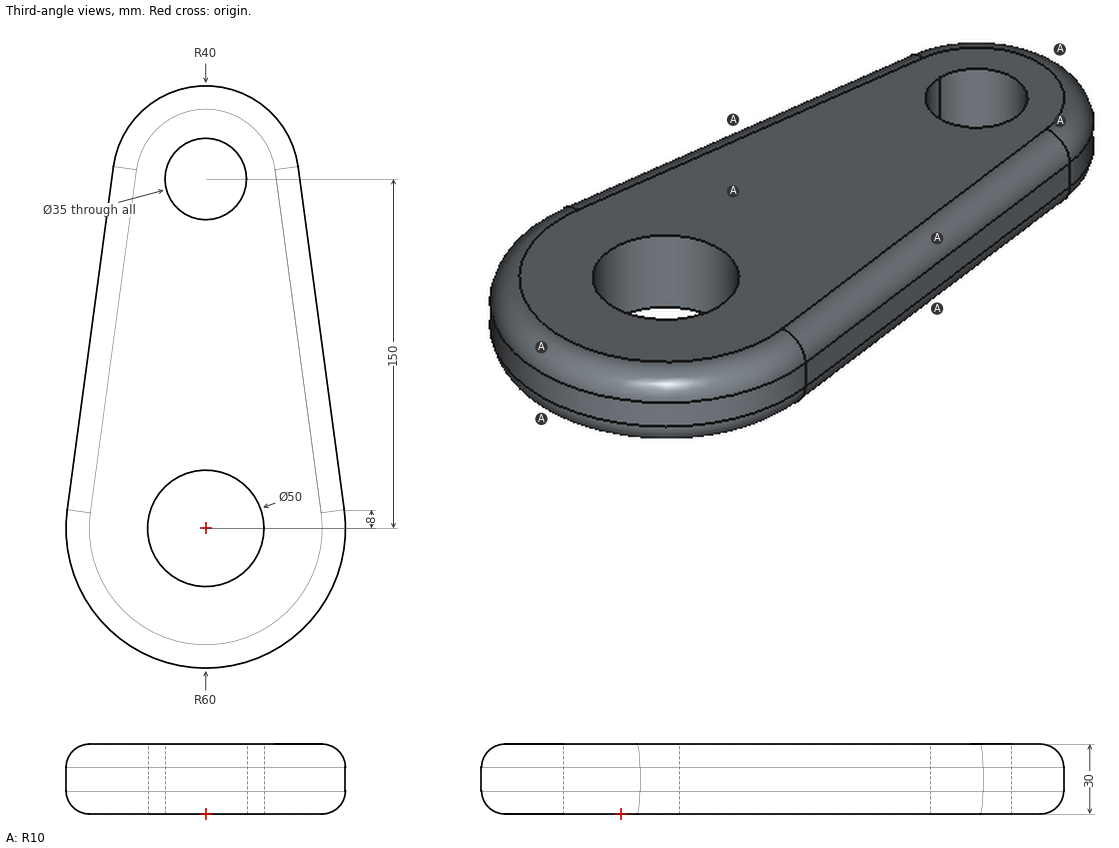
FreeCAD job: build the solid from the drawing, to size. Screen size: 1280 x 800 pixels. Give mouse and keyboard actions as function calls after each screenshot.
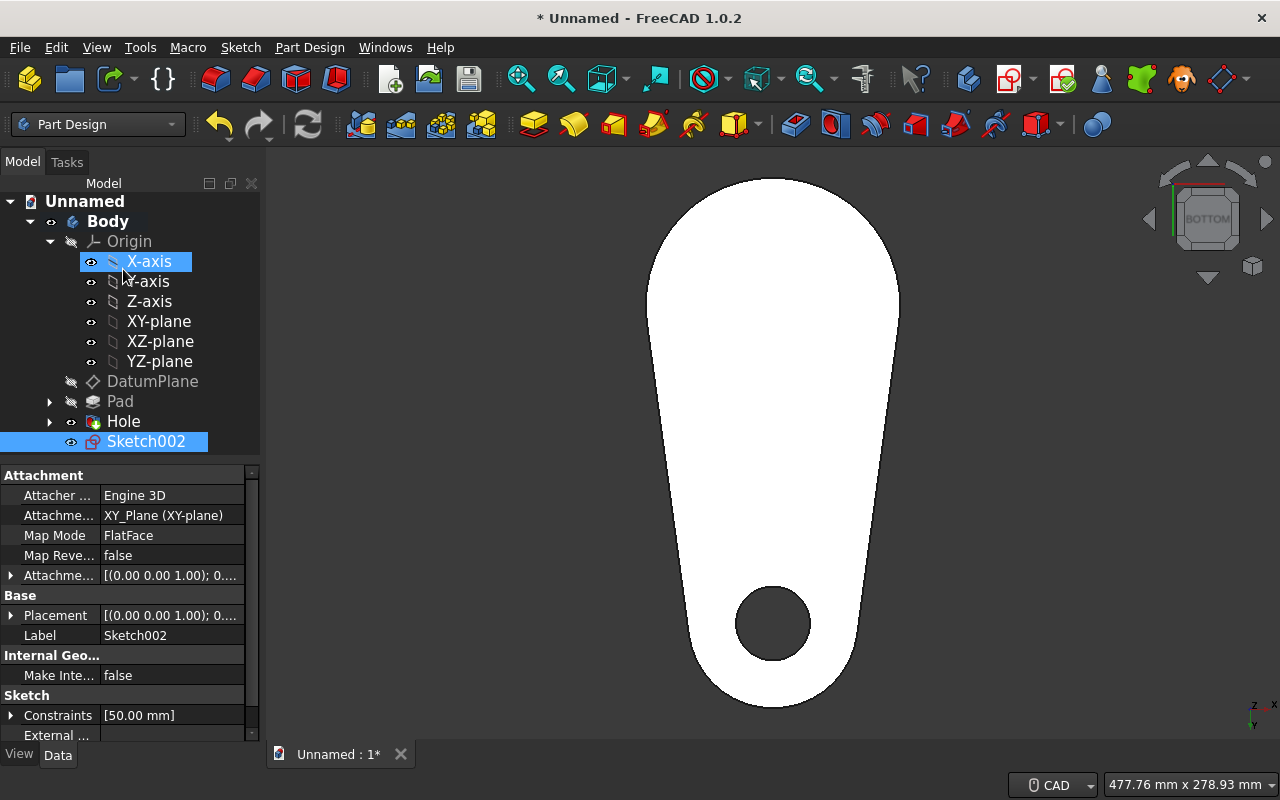
click(796, 124)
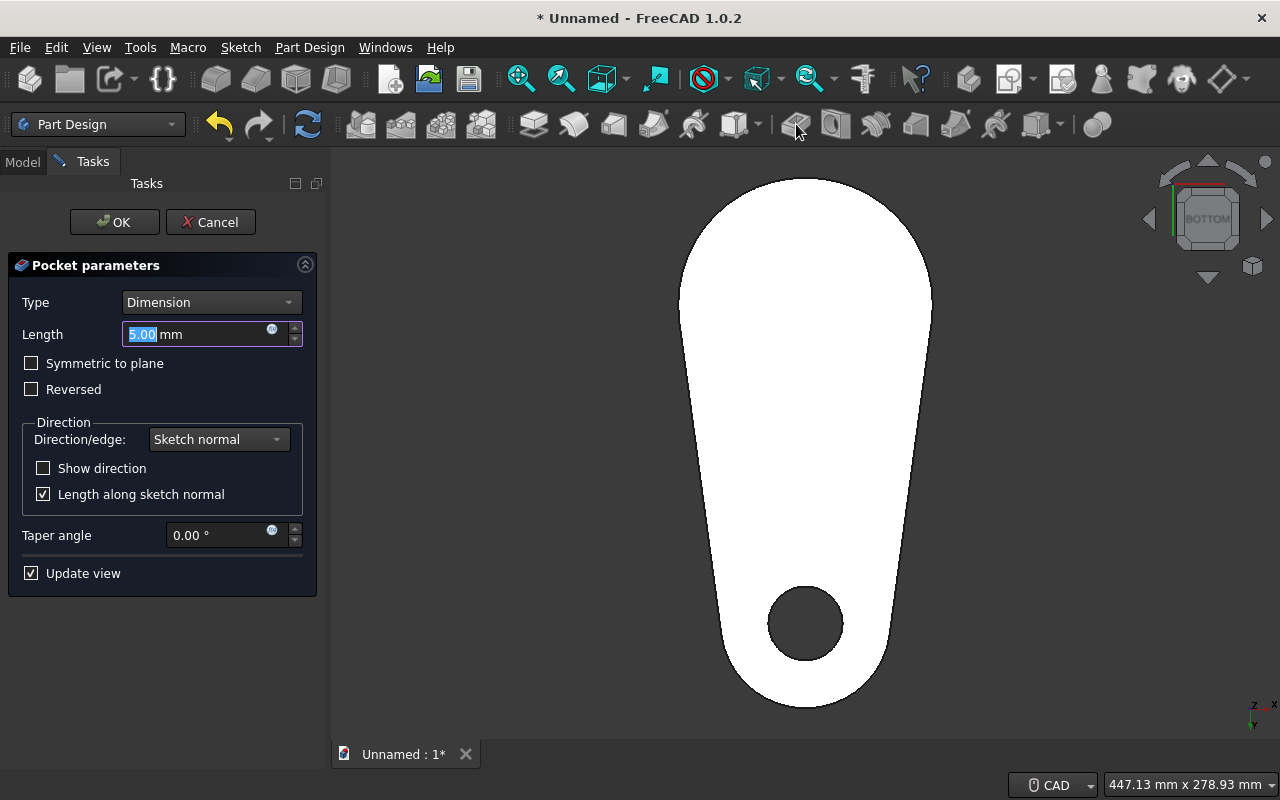
click(212, 302)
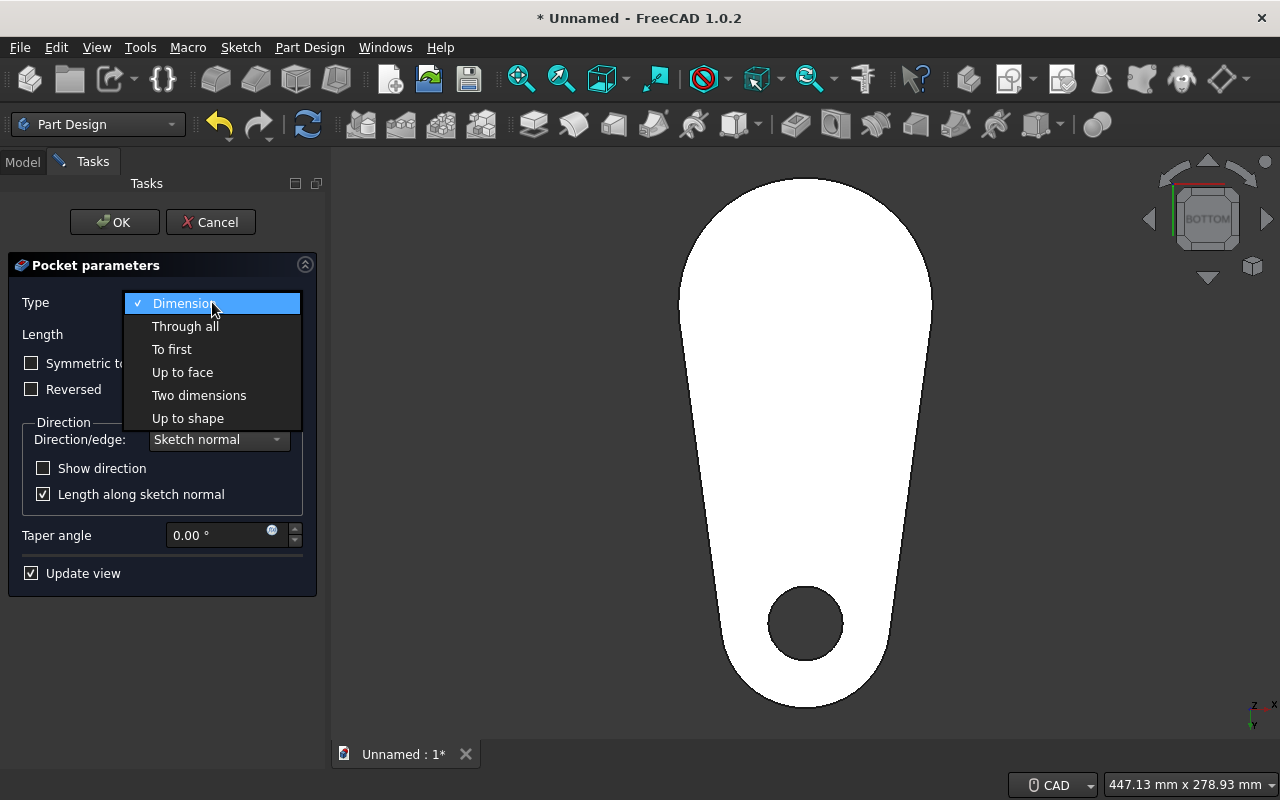
click(212, 326)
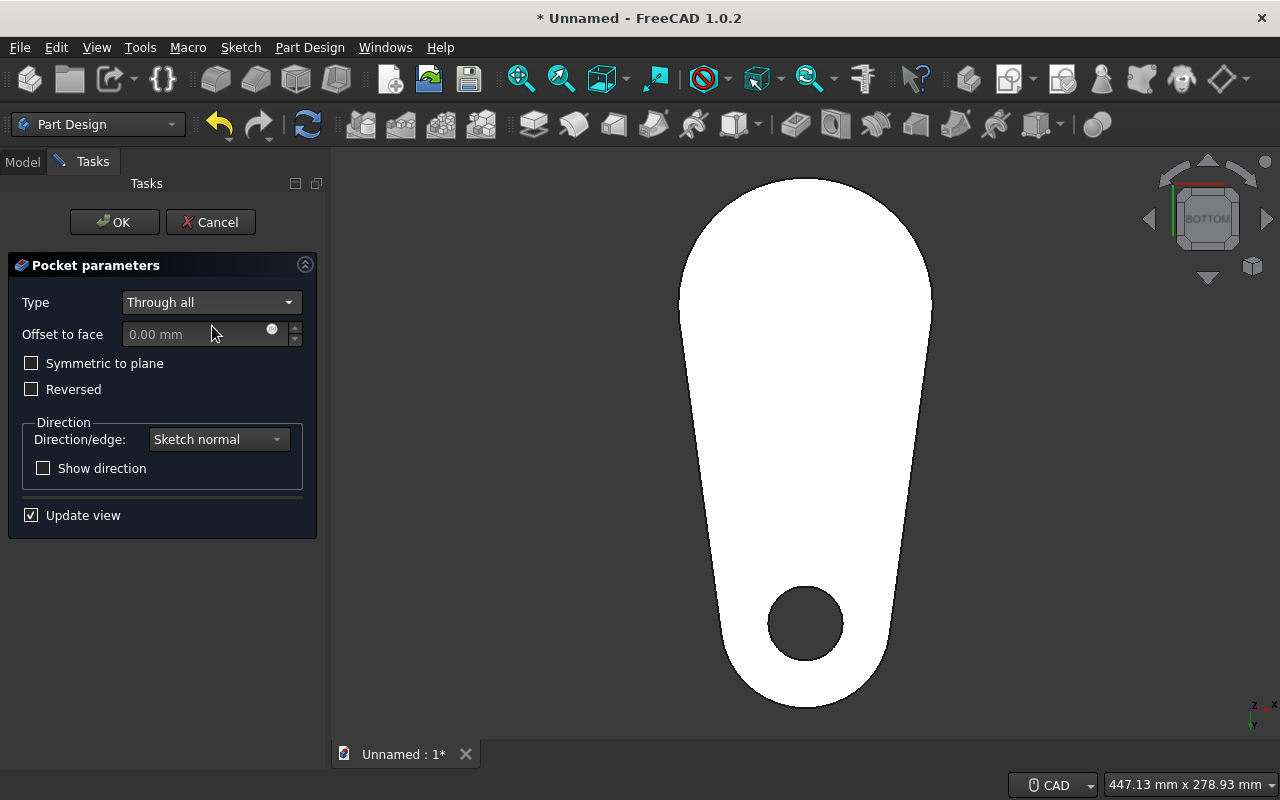
click(30, 389)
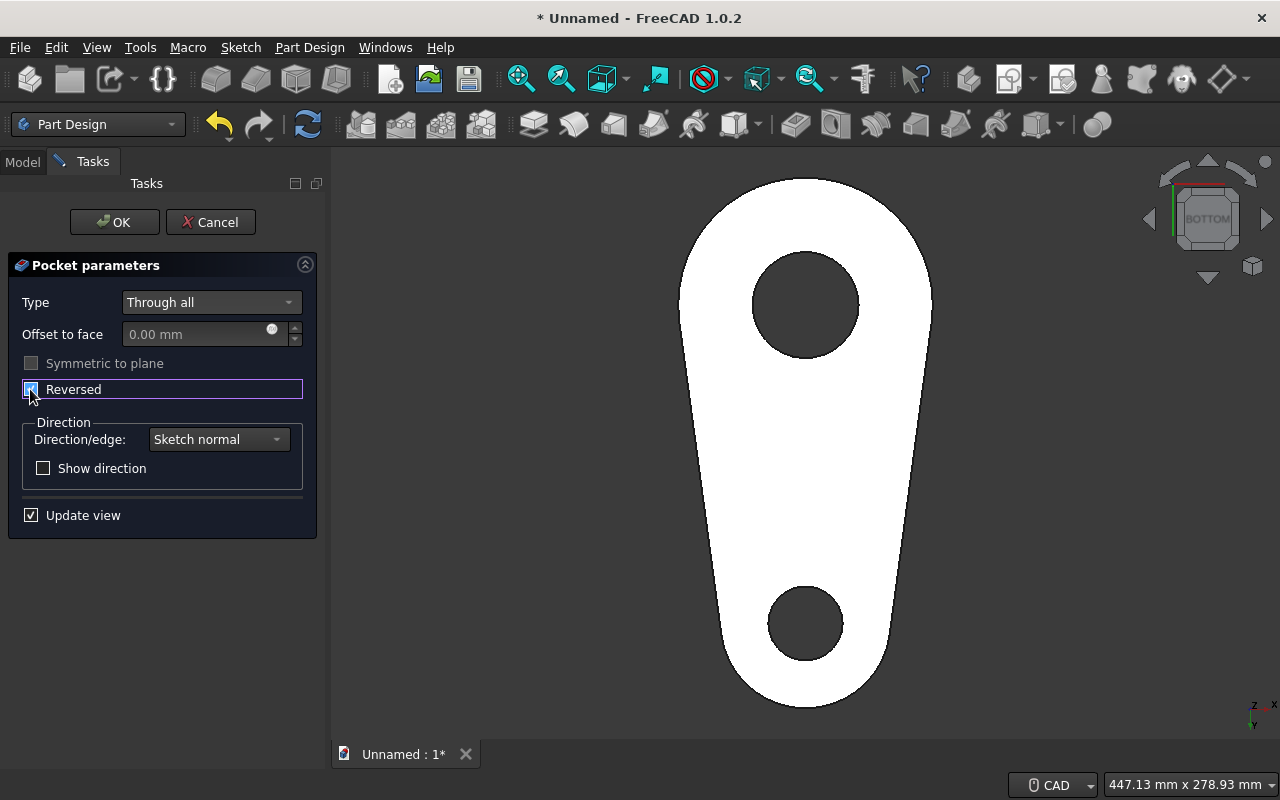
click(115, 222)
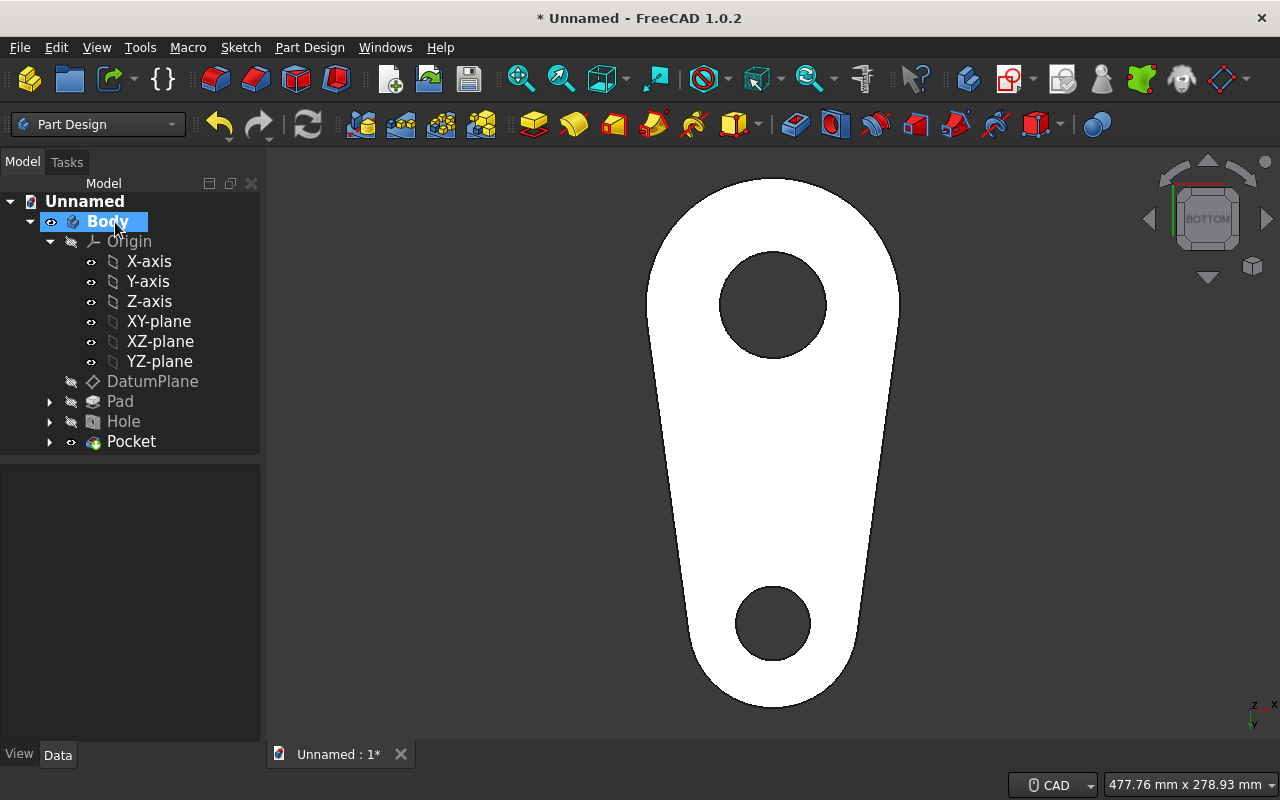
click(773, 707)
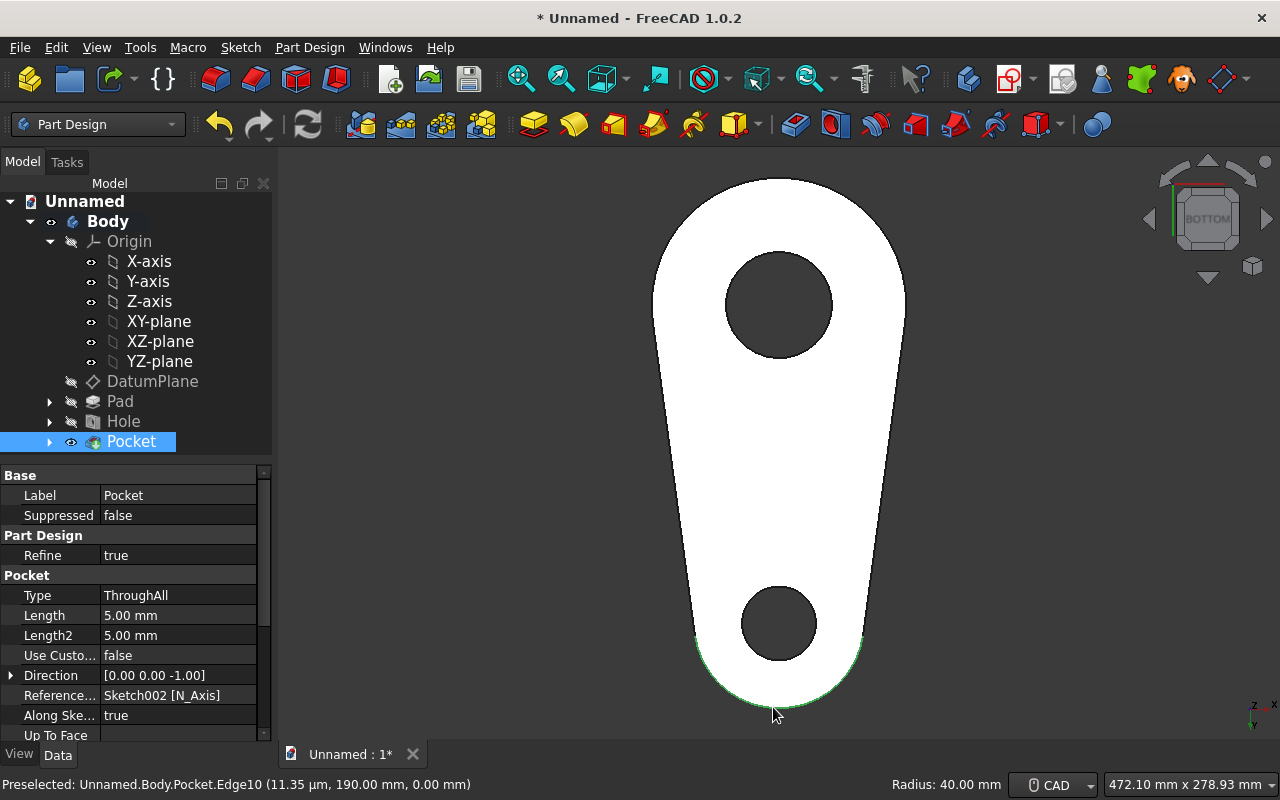
click(674, 477, ctrl)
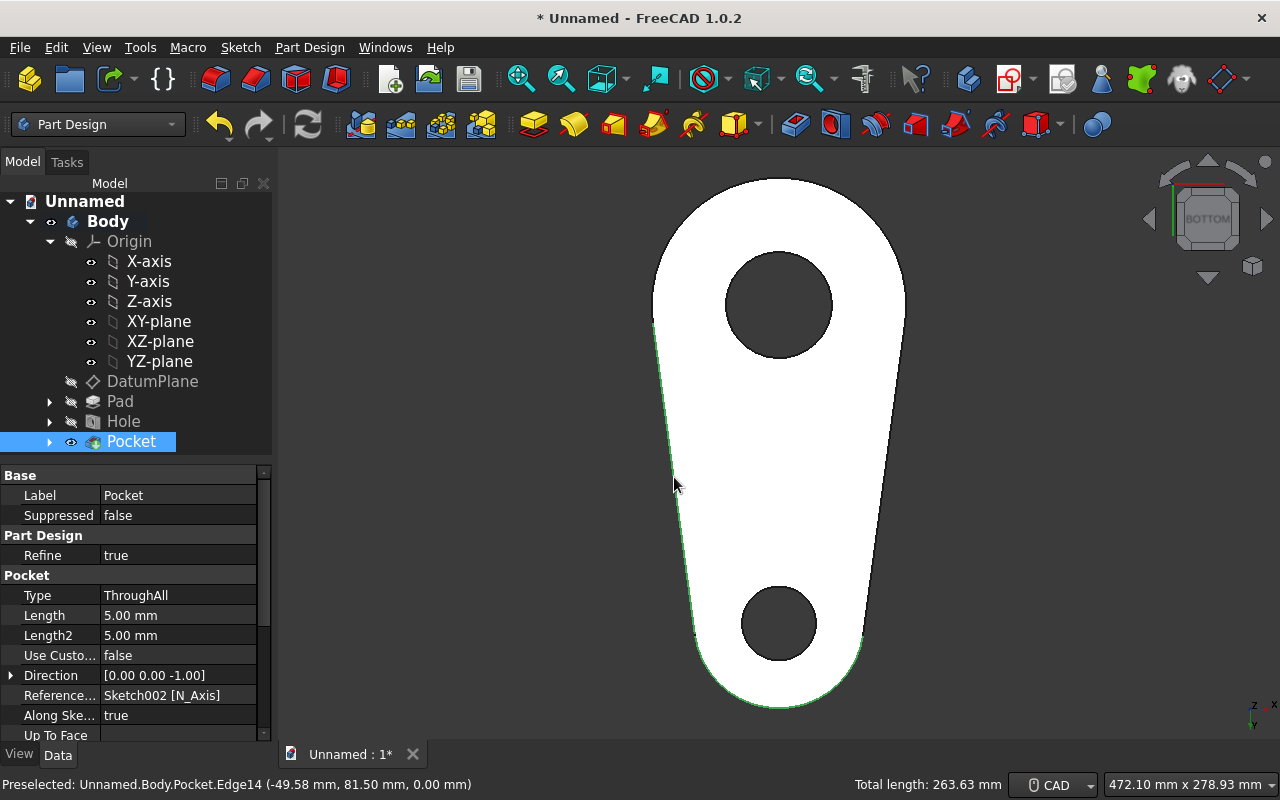
click(670, 238, ctrl)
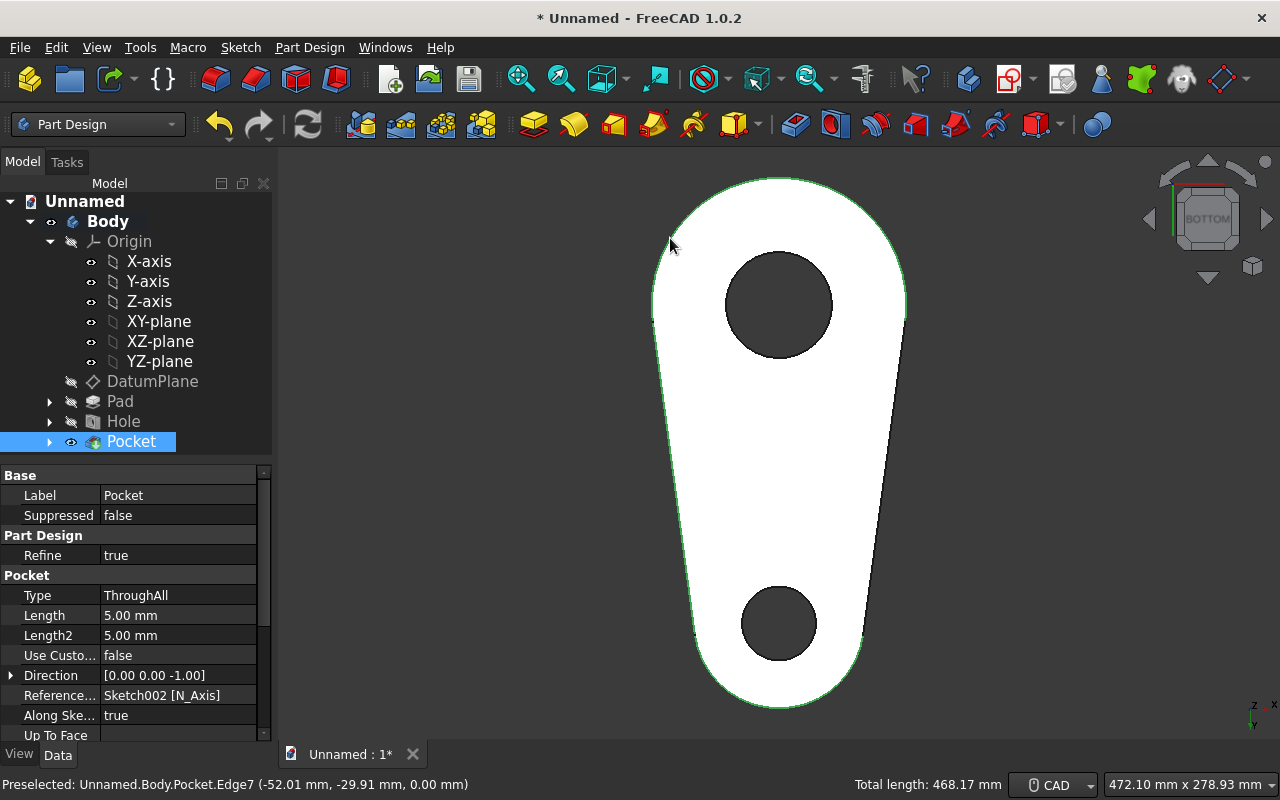
click(884, 477, ctrl)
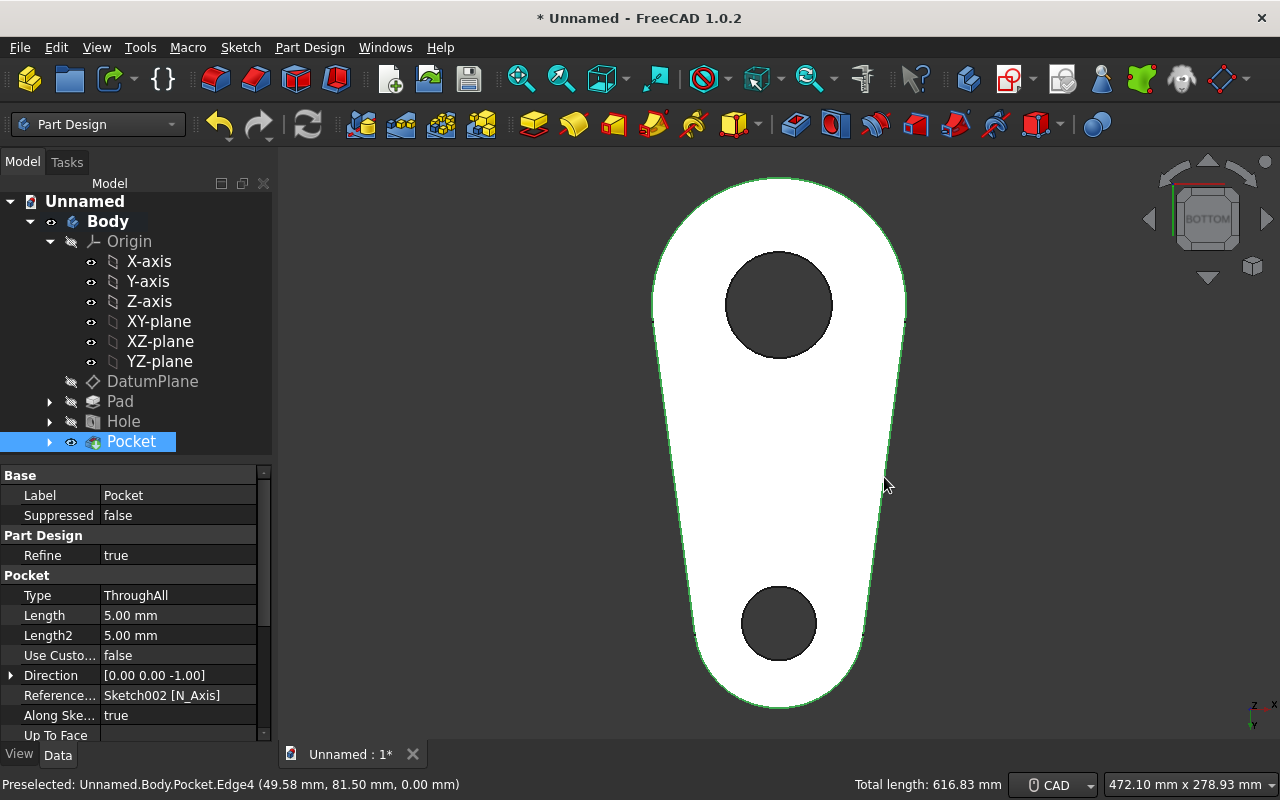
key(0)